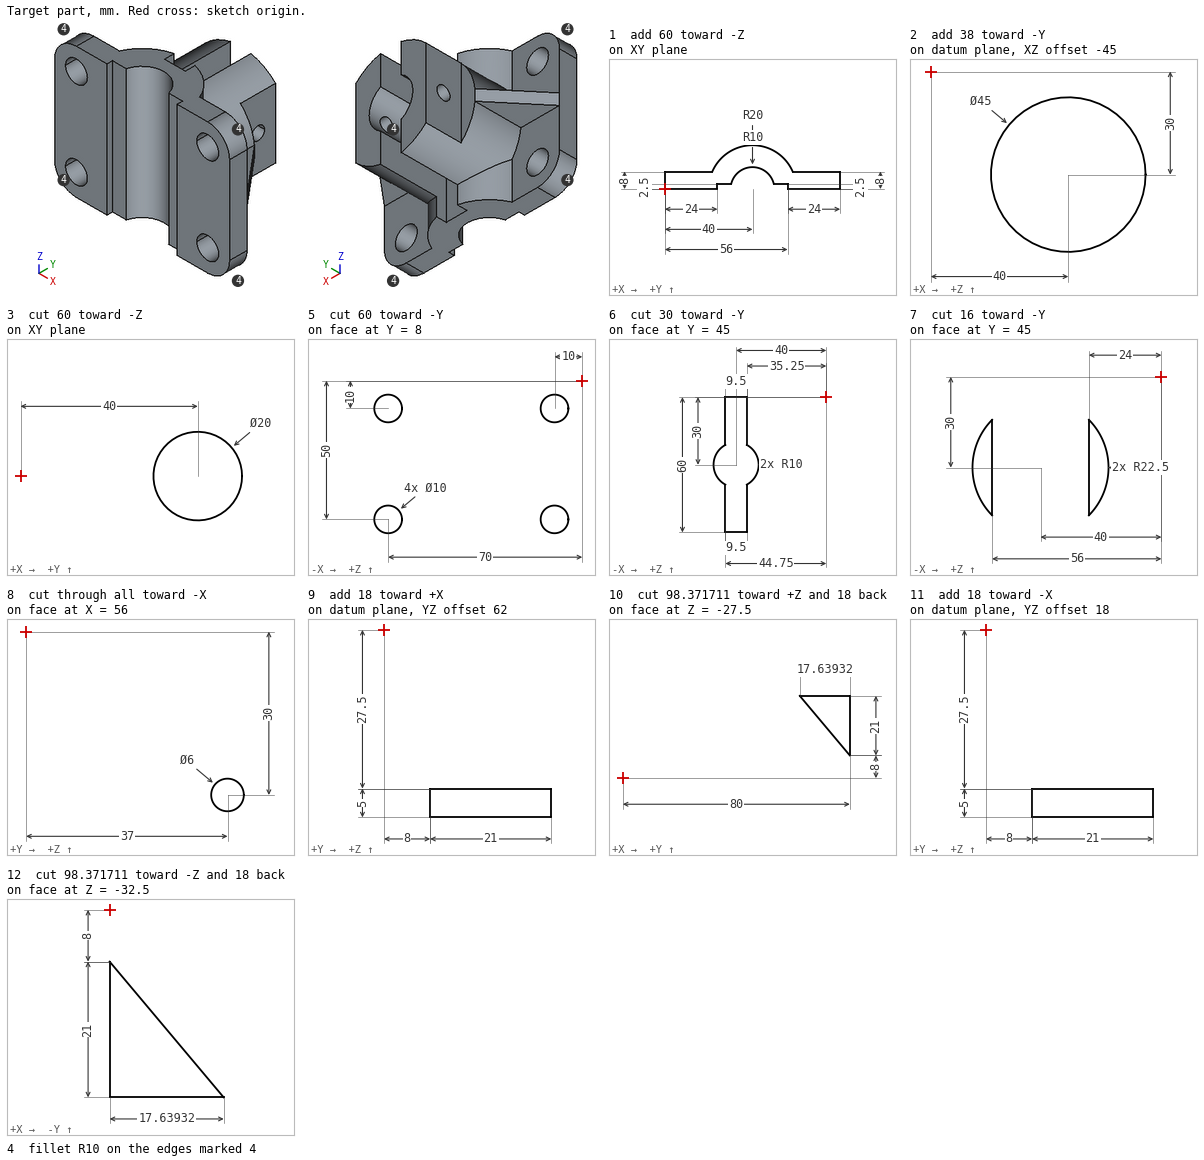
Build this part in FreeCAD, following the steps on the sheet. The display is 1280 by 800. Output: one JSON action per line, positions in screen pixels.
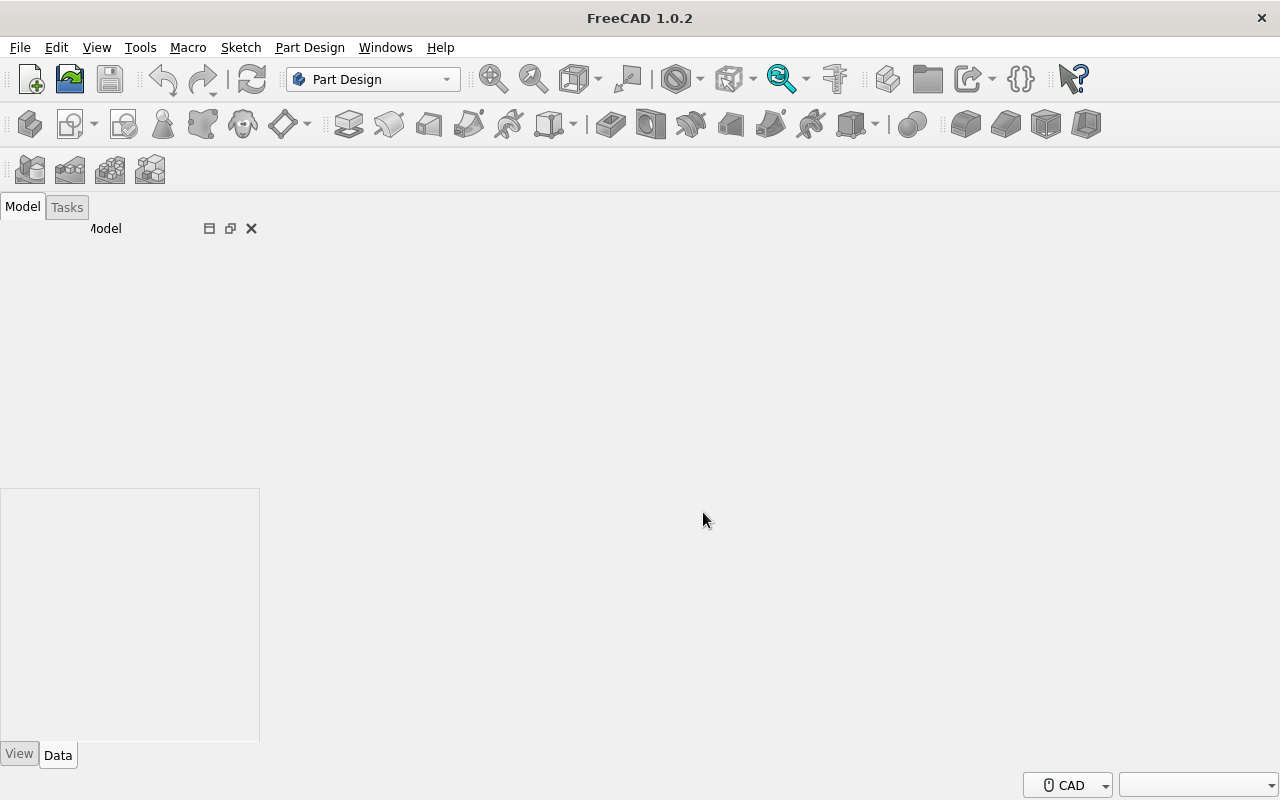
{"action": "left_click", "coordinate": [30, 80]}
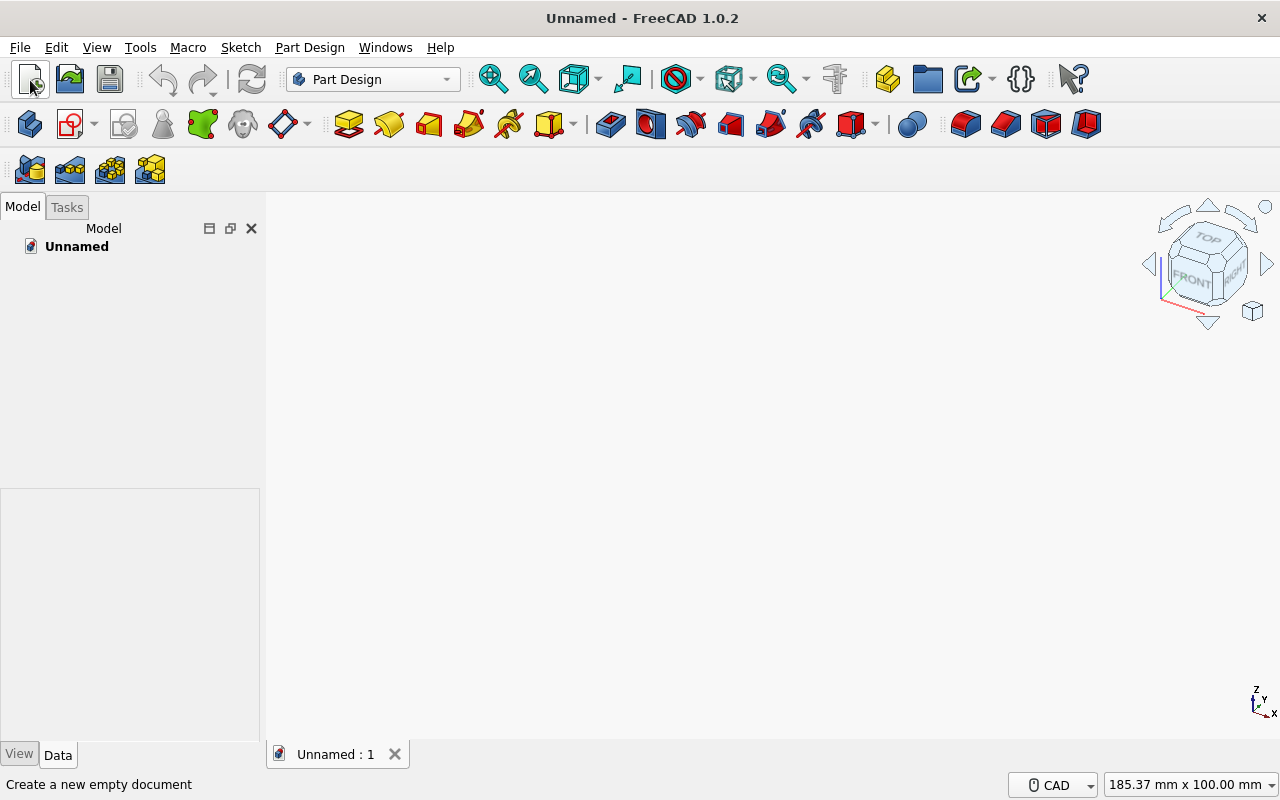
{"action": "left_click", "coordinate": [70, 124]}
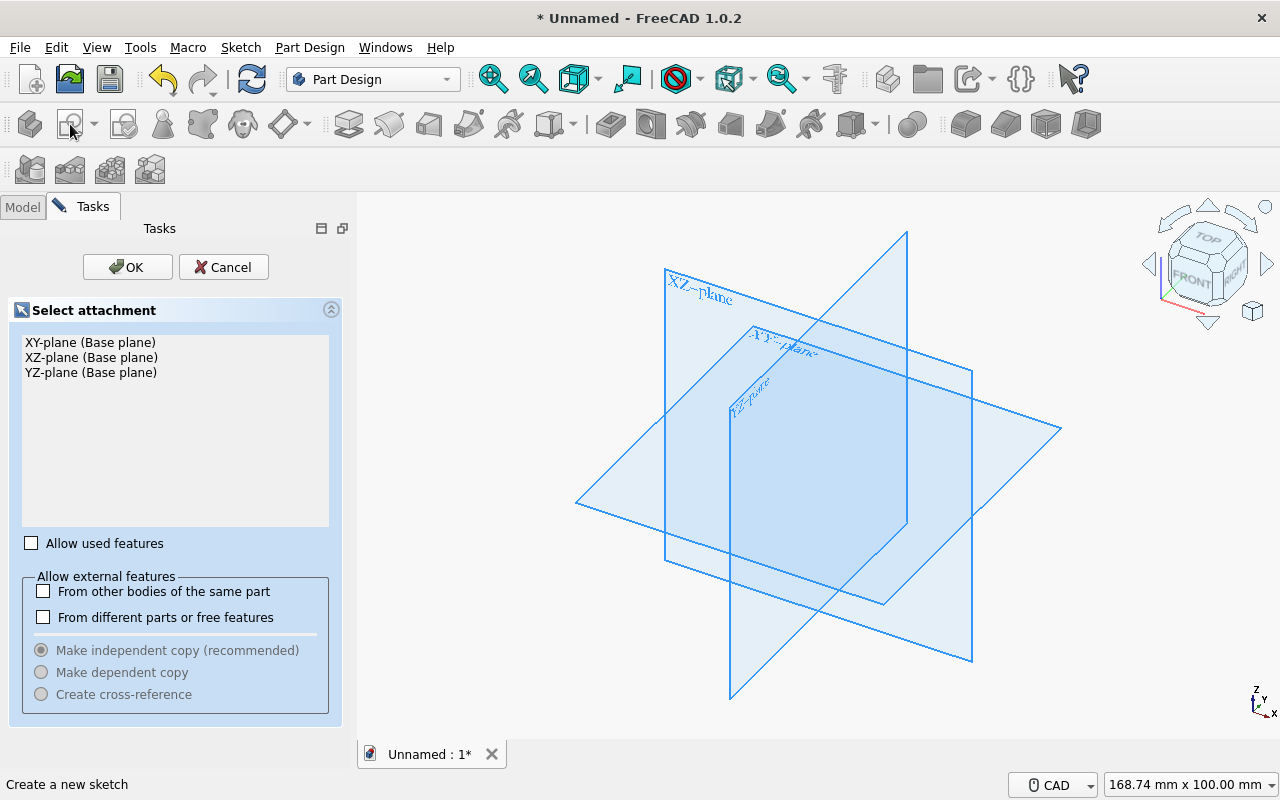
{"action": "left_click", "coordinate": [82, 342]}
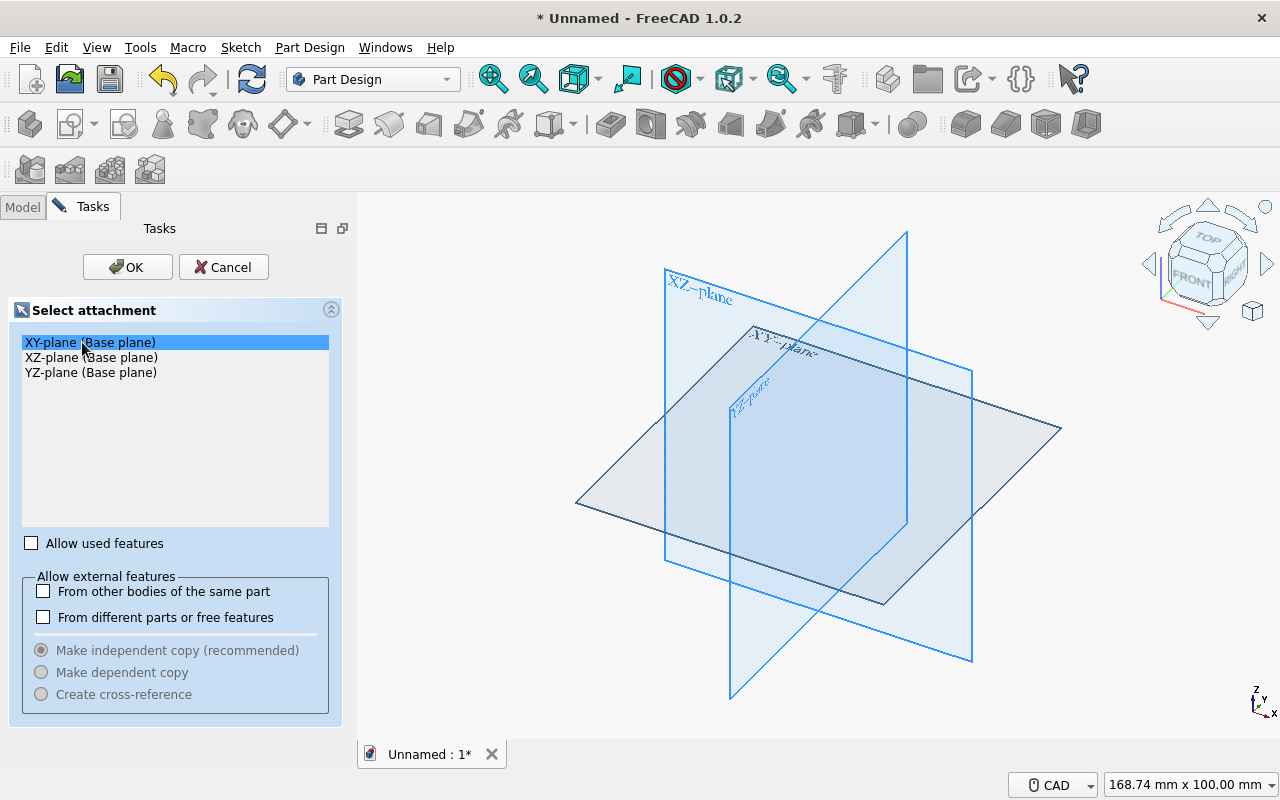
{"action": "left_click", "coordinate": [128, 267]}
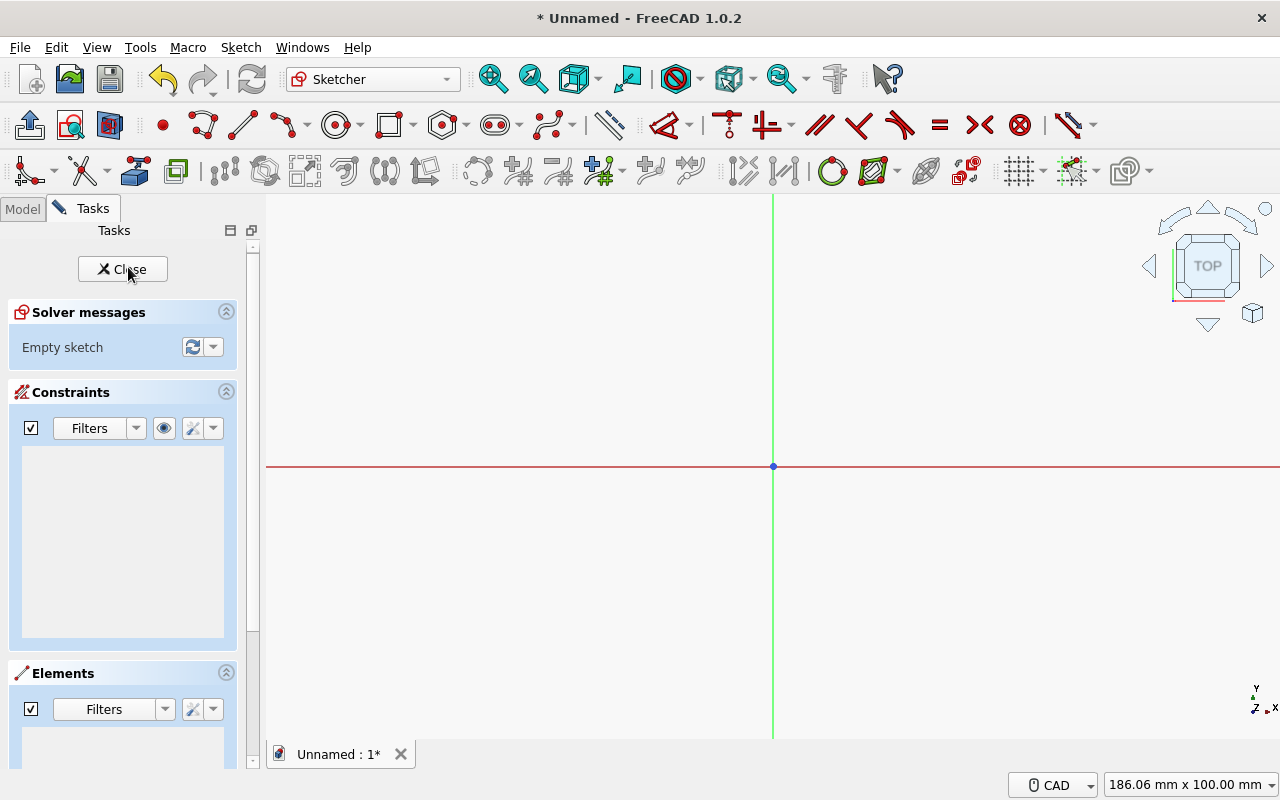
{"action": "scroll", "coordinate": [294, 711], "scroll_direction": "down", "scroll_amount": 1}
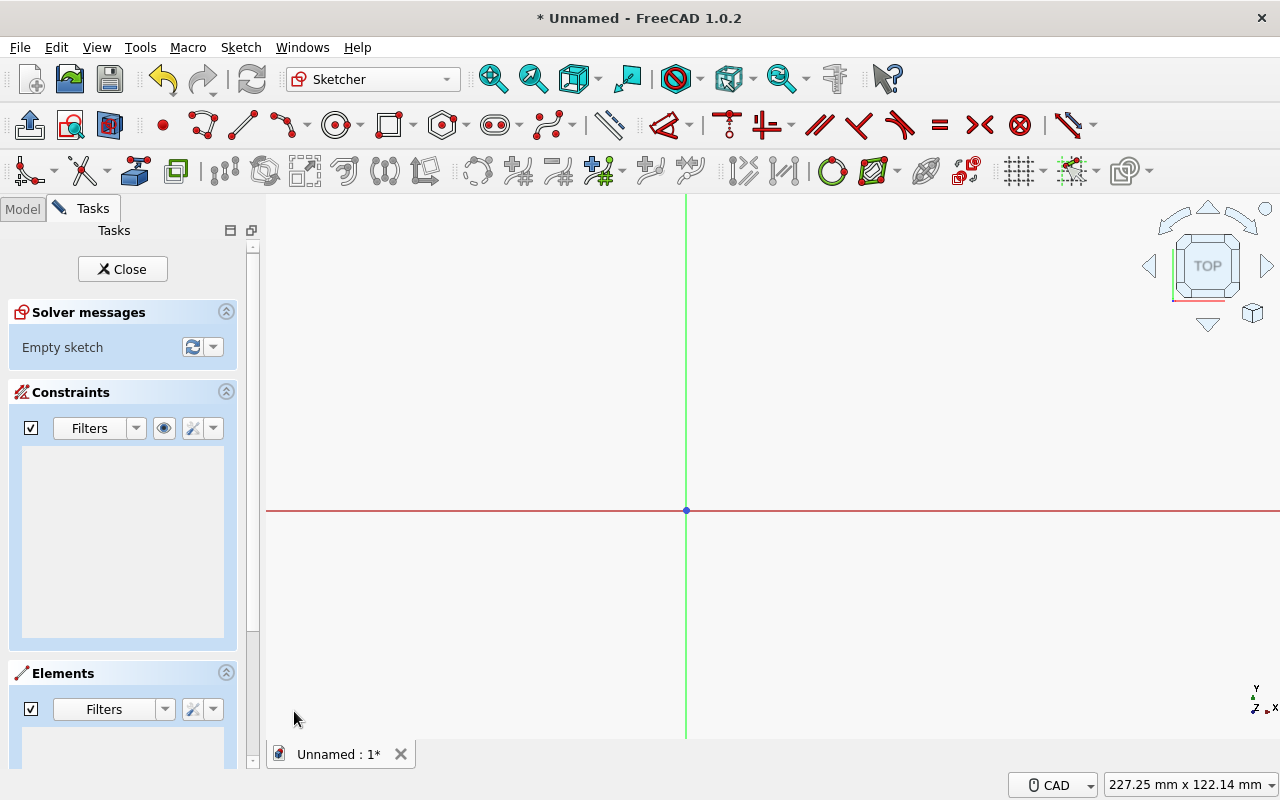
{"action": "scroll", "coordinate": [1115, 466], "scroll_direction": "up", "scroll_amount": 2}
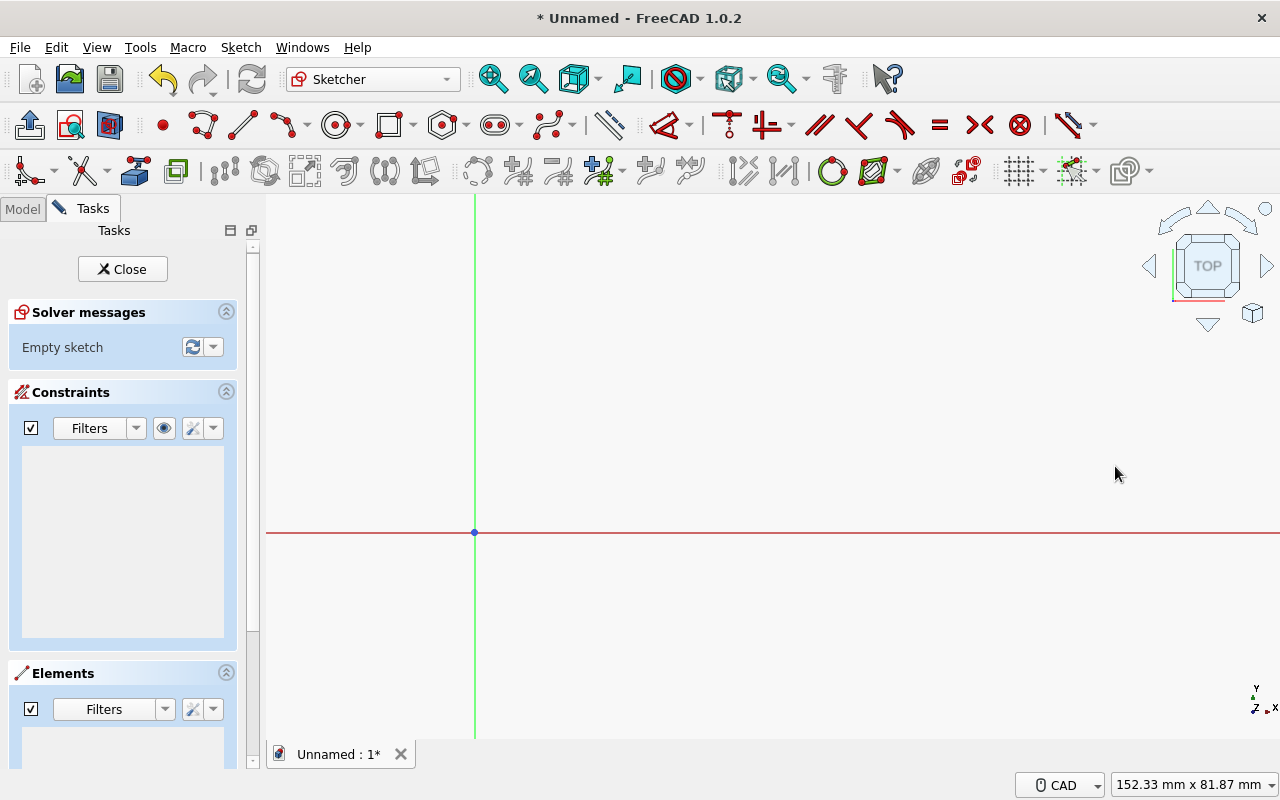
{"action": "left_click", "coordinate": [204, 126]}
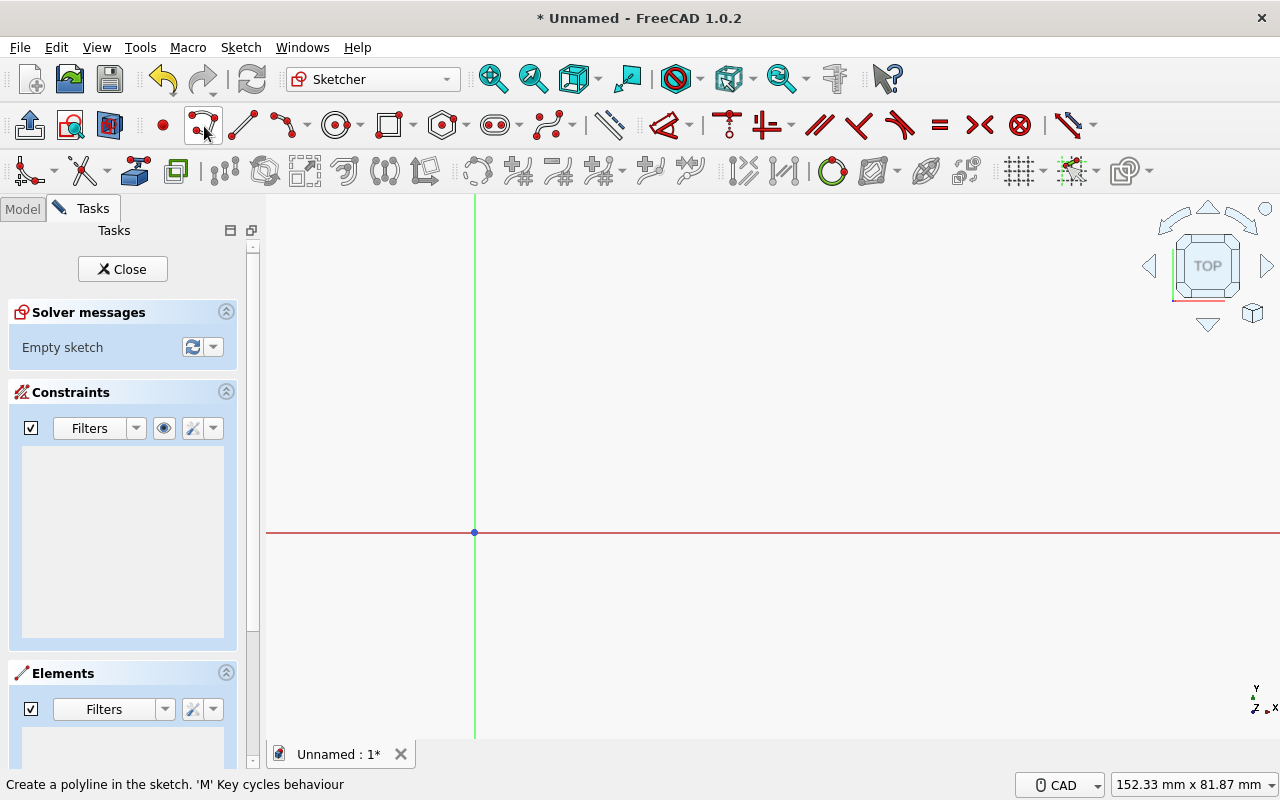
{"action": "left_click", "coordinate": [806, 516]}
{"action": "left_click", "coordinate": [848, 516]}
{"action": "left_click", "coordinate": [848, 533]}
{"action": "left_click", "coordinate": [1007, 524]}
{"action": "left_click", "coordinate": [1007, 480]}
{"action": "left_click", "coordinate": [863, 480]}
{"action": "right_click", "coordinate": [863, 480]}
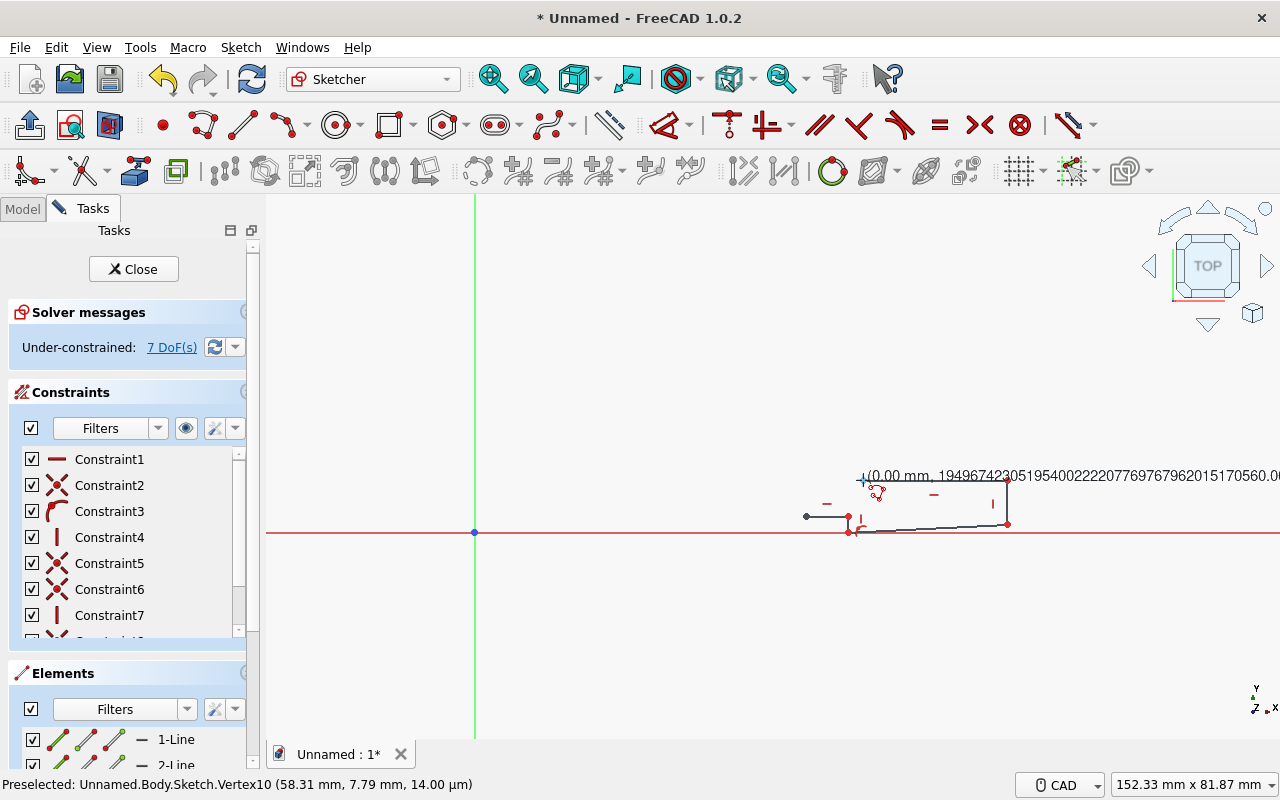
{"action": "left_click", "coordinate": [619, 480]}
{"action": "left_click", "coordinate": [475, 480]}
{"action": "left_click", "coordinate": [475, 533]}
{"action": "left_click", "coordinate": [635, 524]}
{"action": "left_click", "coordinate": [635, 516]}
{"action": "left_click", "coordinate": [677, 516]}
{"action": "right_click", "coordinate": [677, 516]}